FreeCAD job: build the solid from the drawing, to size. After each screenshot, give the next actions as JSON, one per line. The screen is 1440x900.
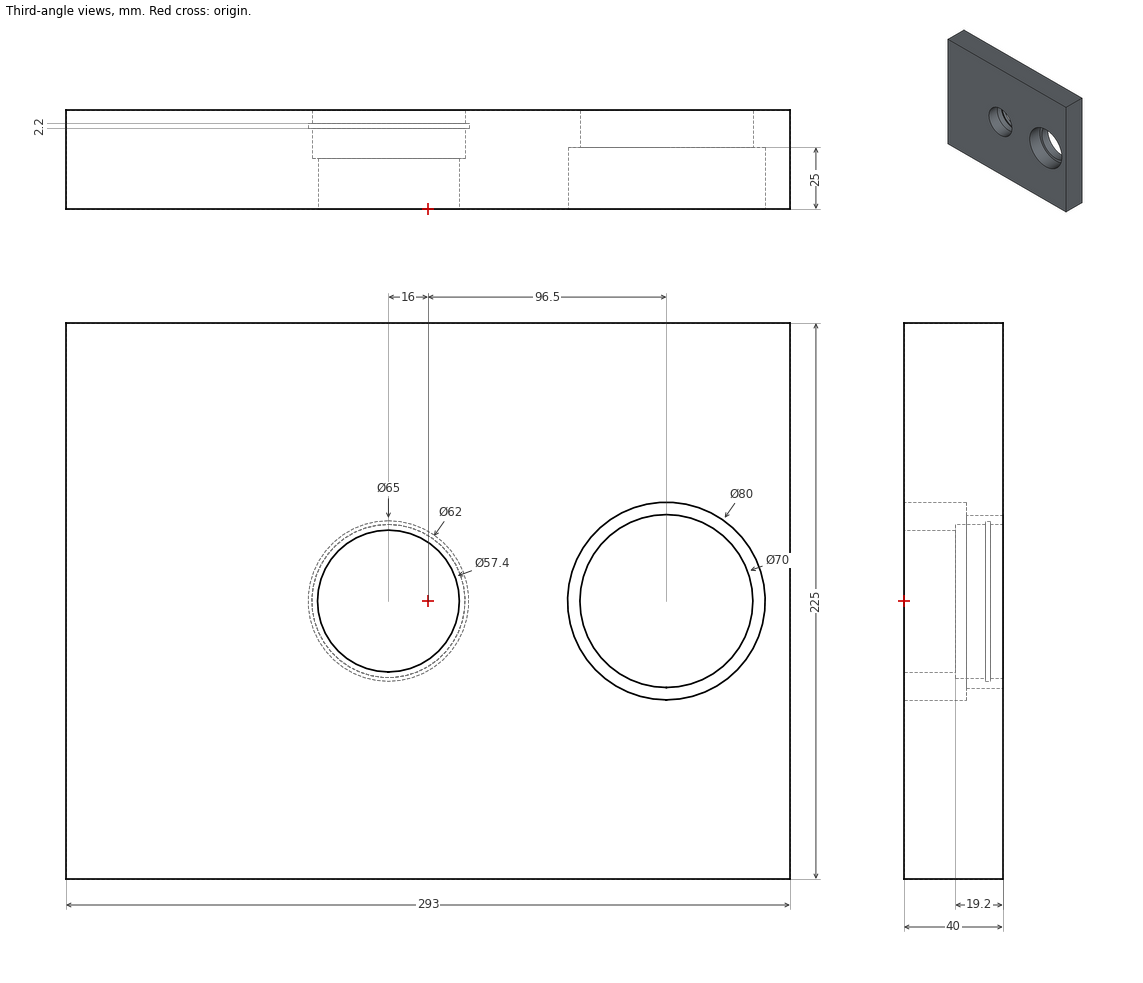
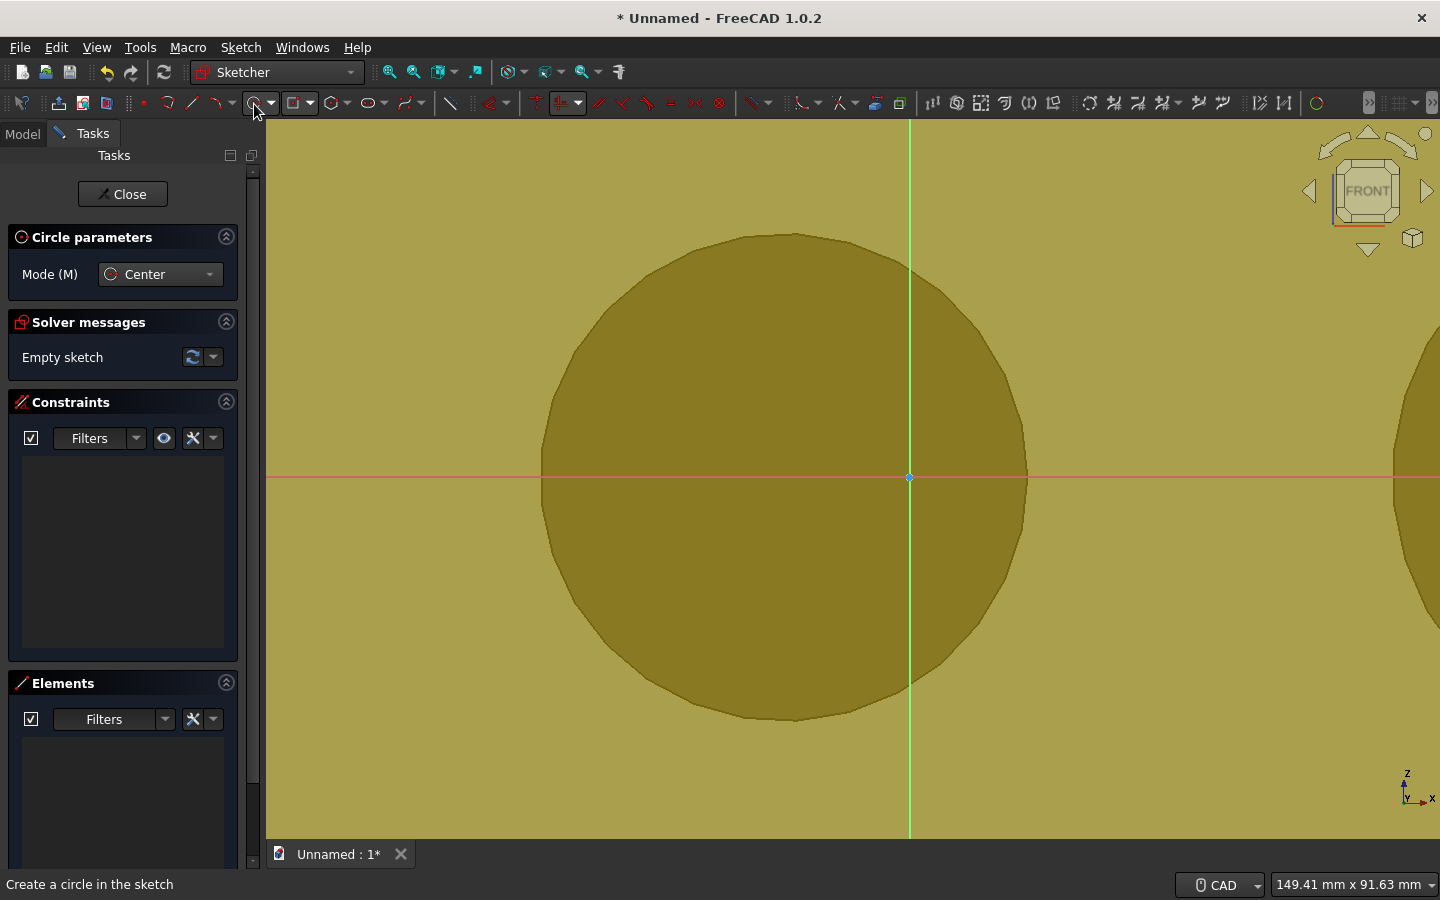
{"action": "left_click", "coordinate": [784, 477]}
{"action": "mouse_move", "coordinate": [964, 297]}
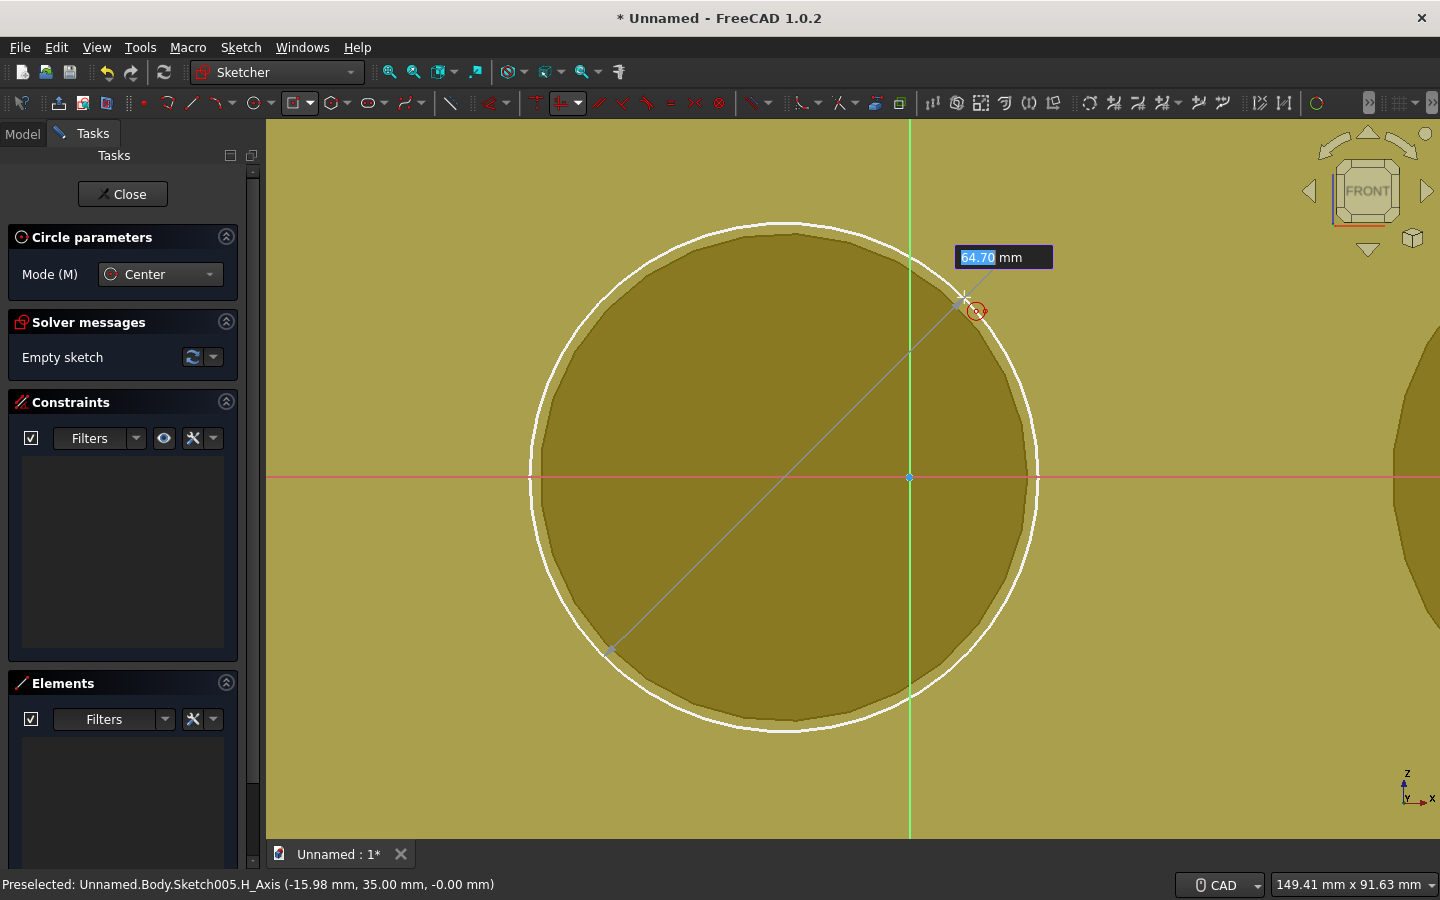
{"action": "type", "text": "65"}
{"action": "key", "text": "Return"}
{"action": "key", "text": "Escape"}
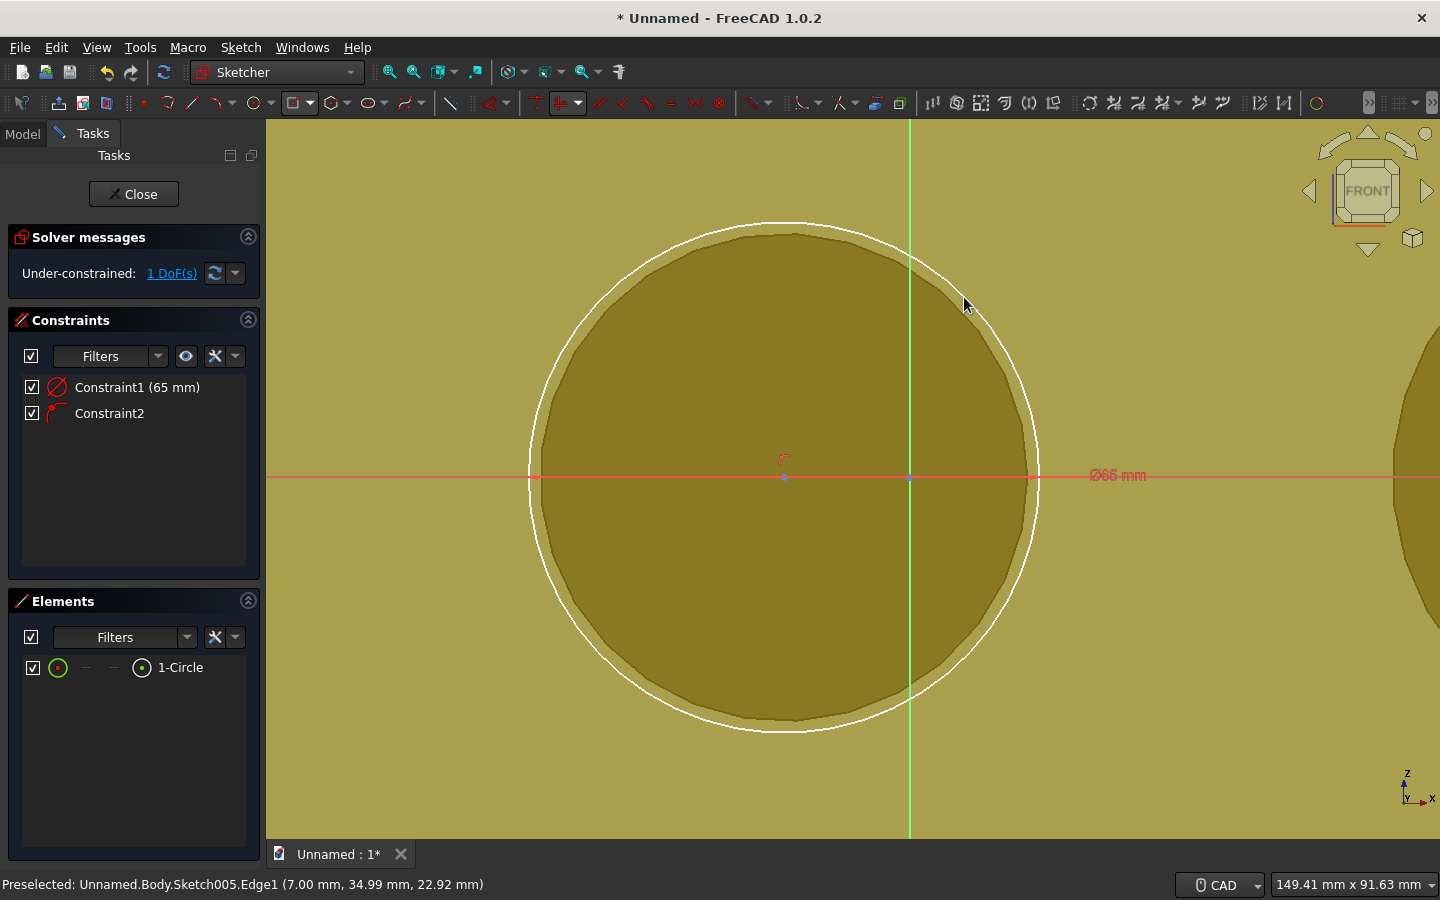
{"action": "left_click", "coordinate": [490, 104]}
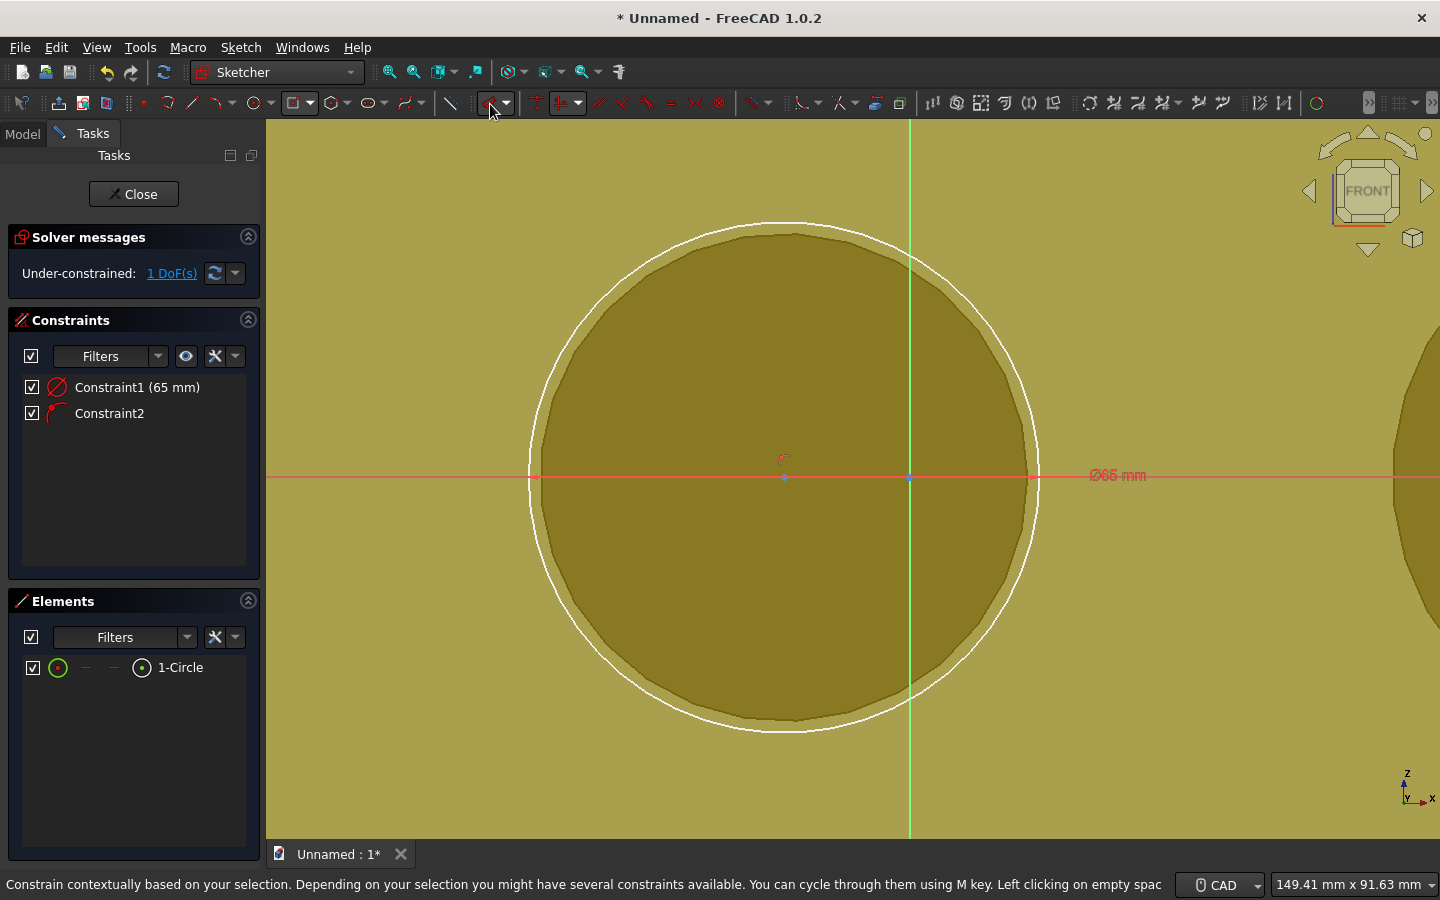
{"action": "left_click", "coordinate": [784, 477]}
{"action": "left_click", "coordinate": [847, 511]}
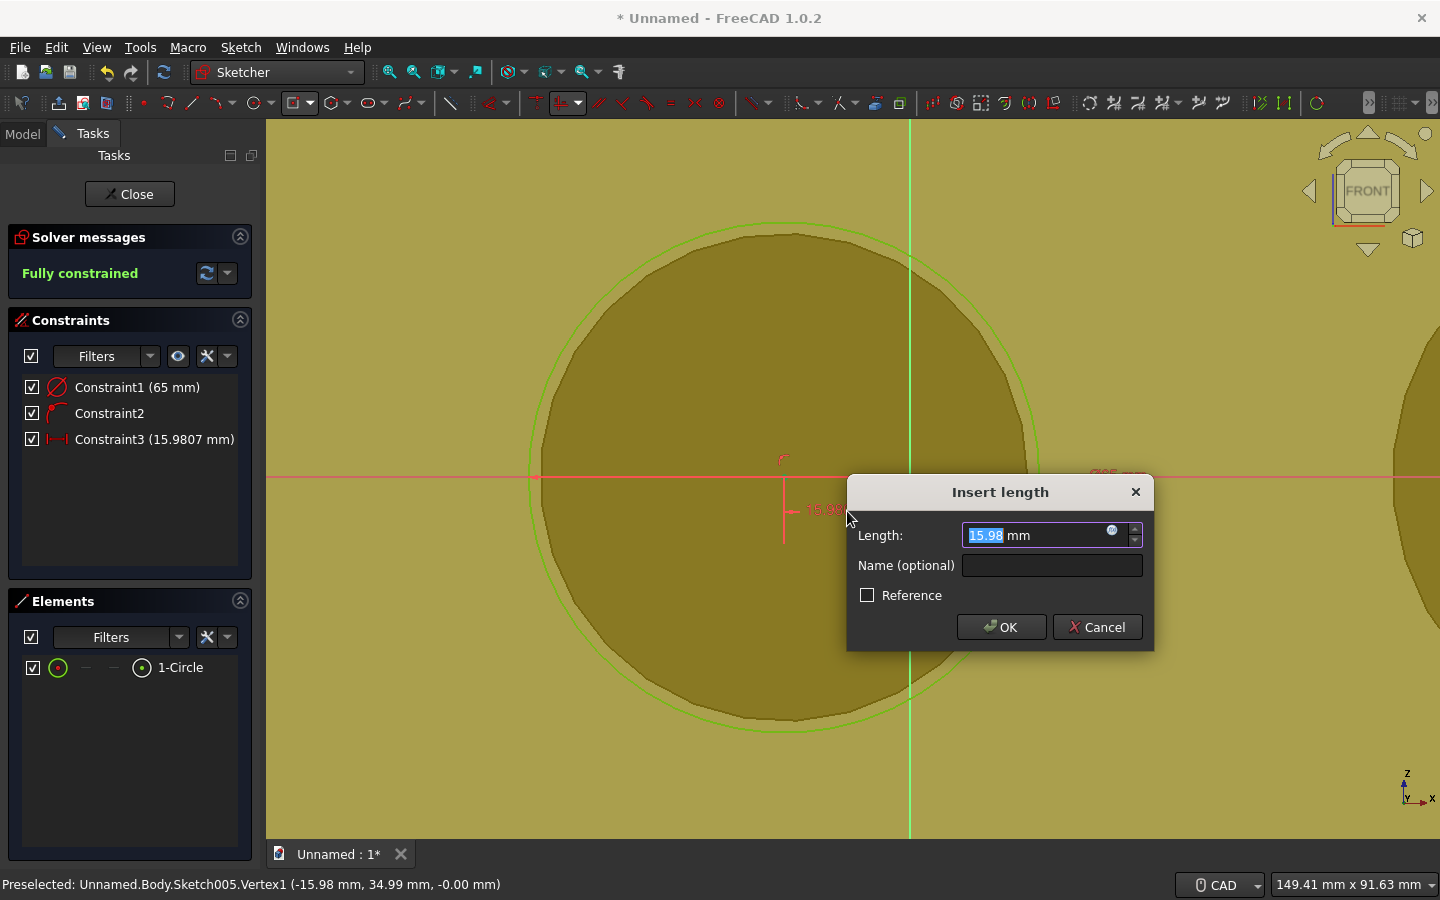
{"action": "type", "text": "16"}
{"action": "key", "text": "Return"}
{"action": "key", "text": "Escape"}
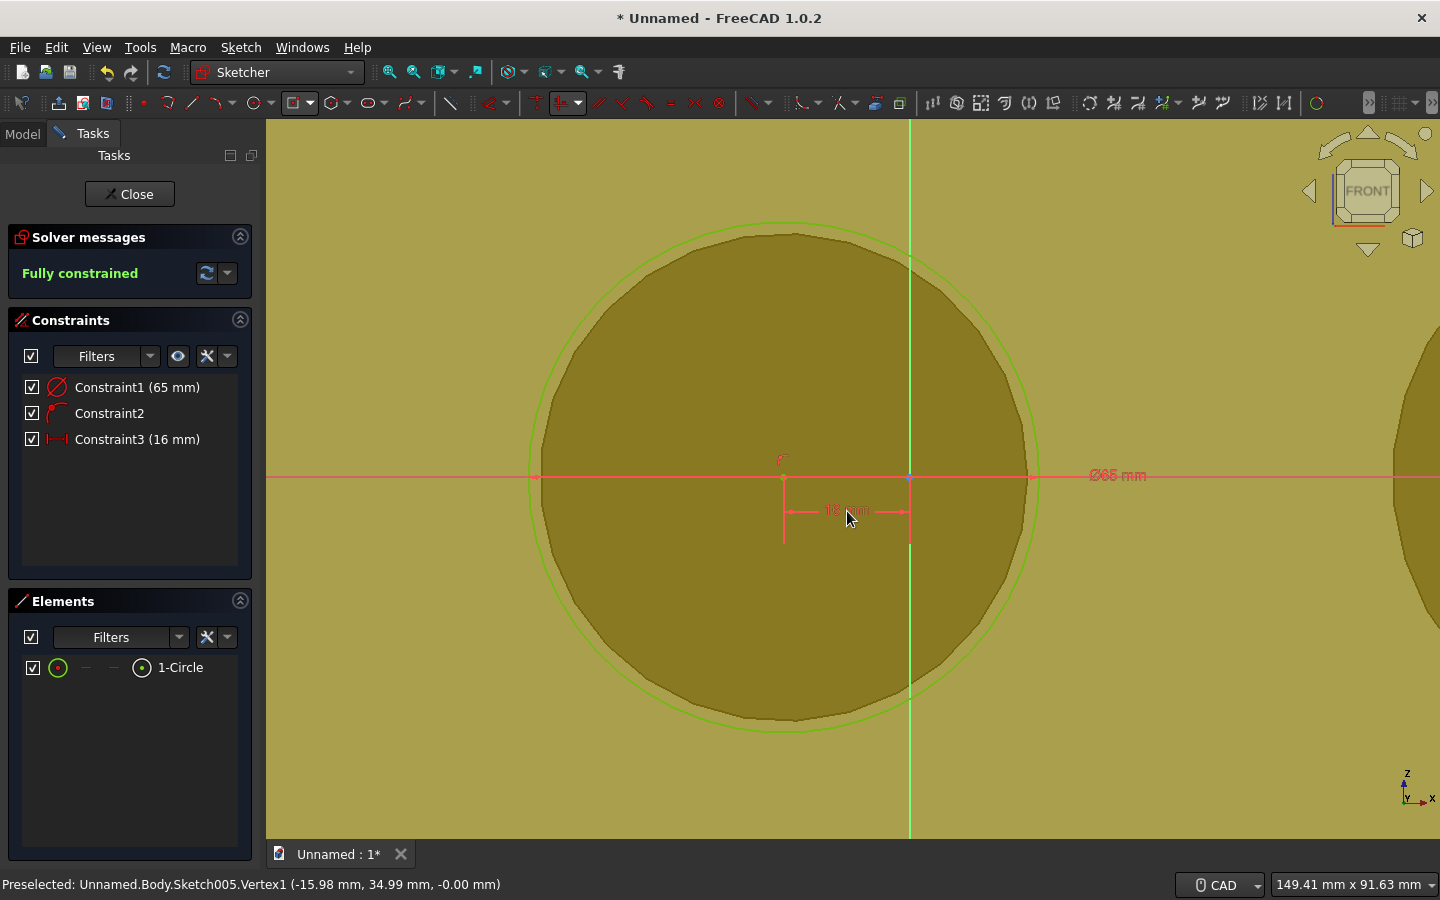
{"action": "left_click", "coordinate": [130, 194]}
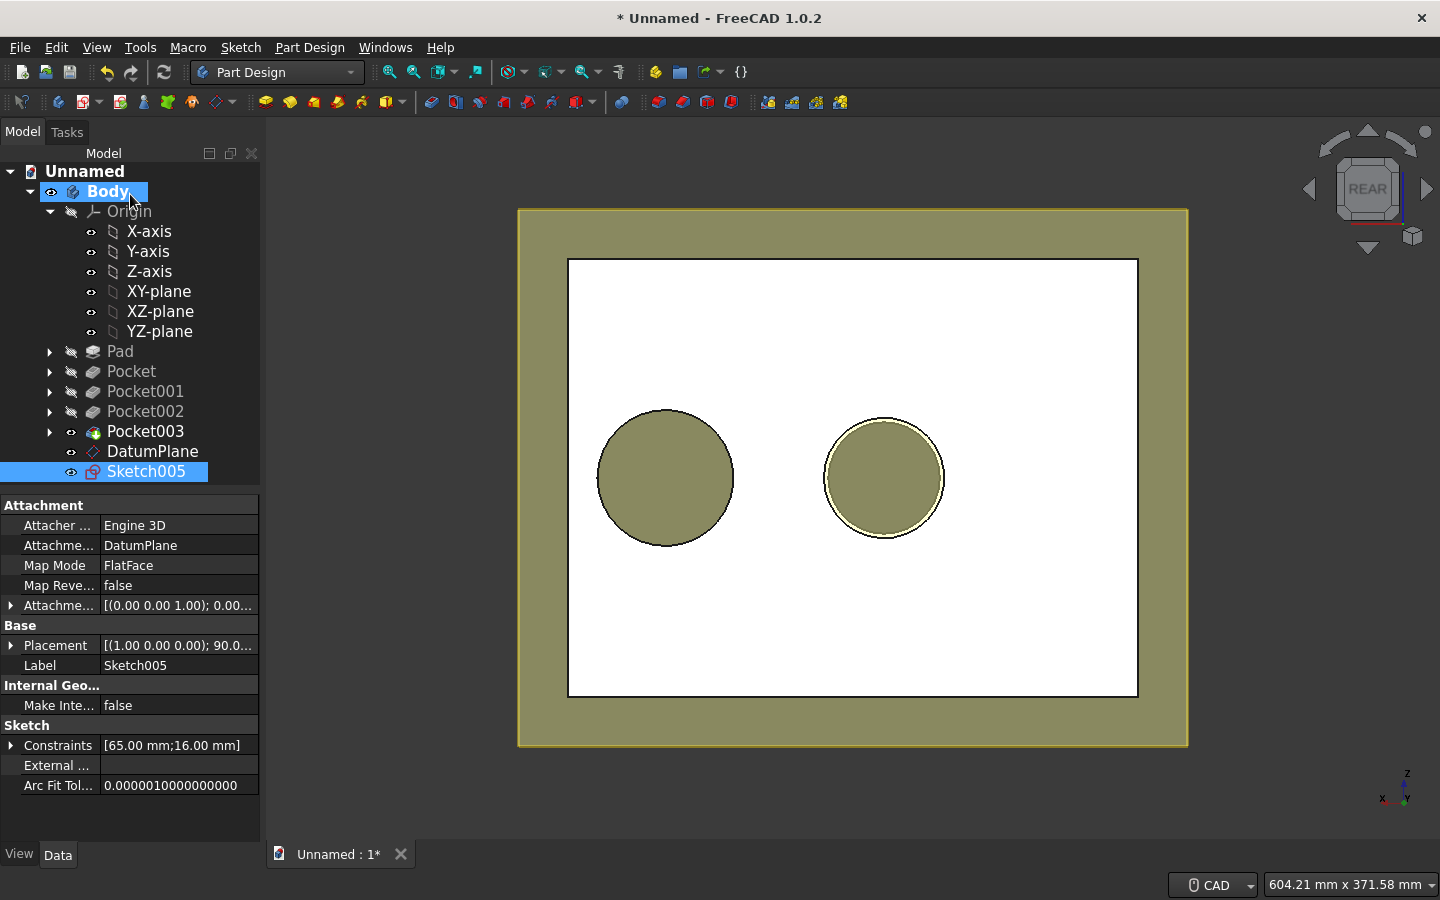
{"action": "left_click", "coordinate": [432, 102]}